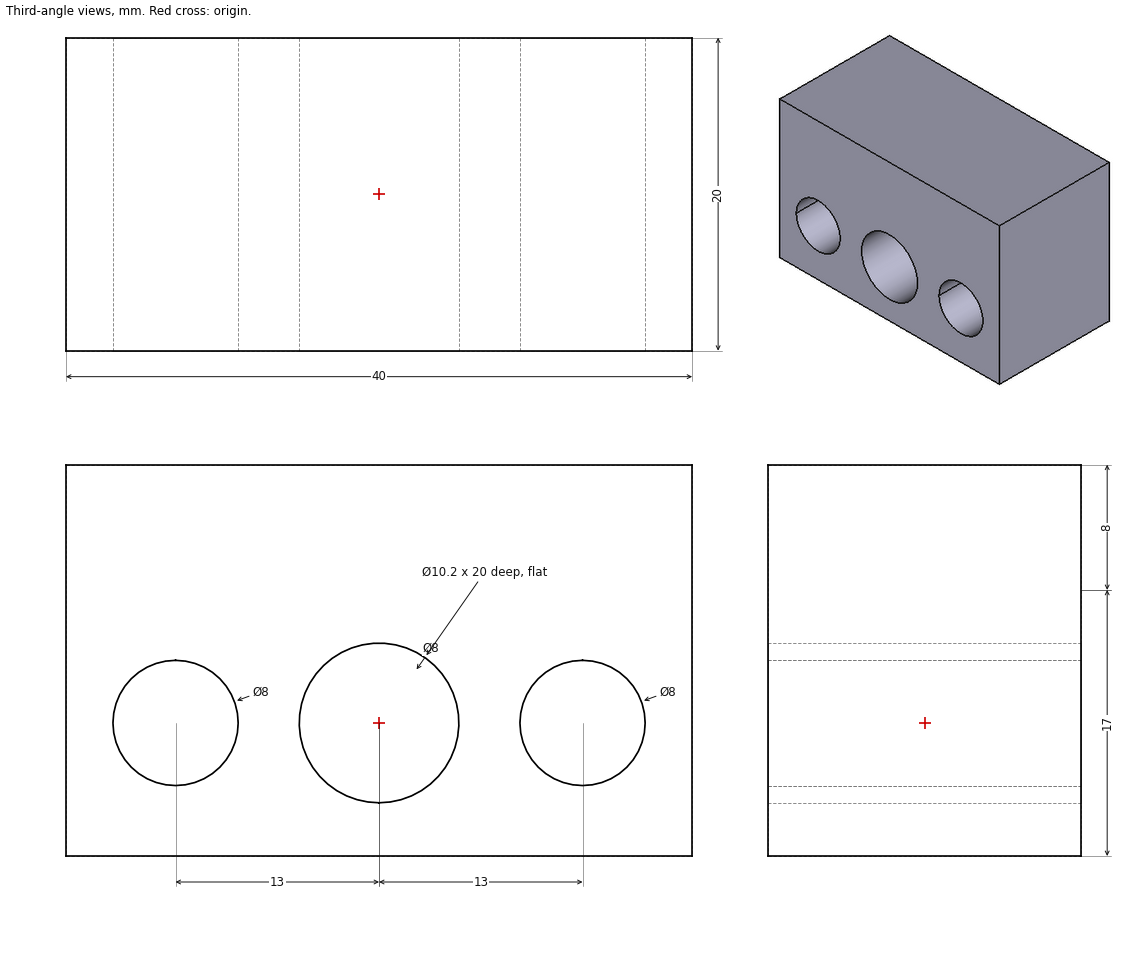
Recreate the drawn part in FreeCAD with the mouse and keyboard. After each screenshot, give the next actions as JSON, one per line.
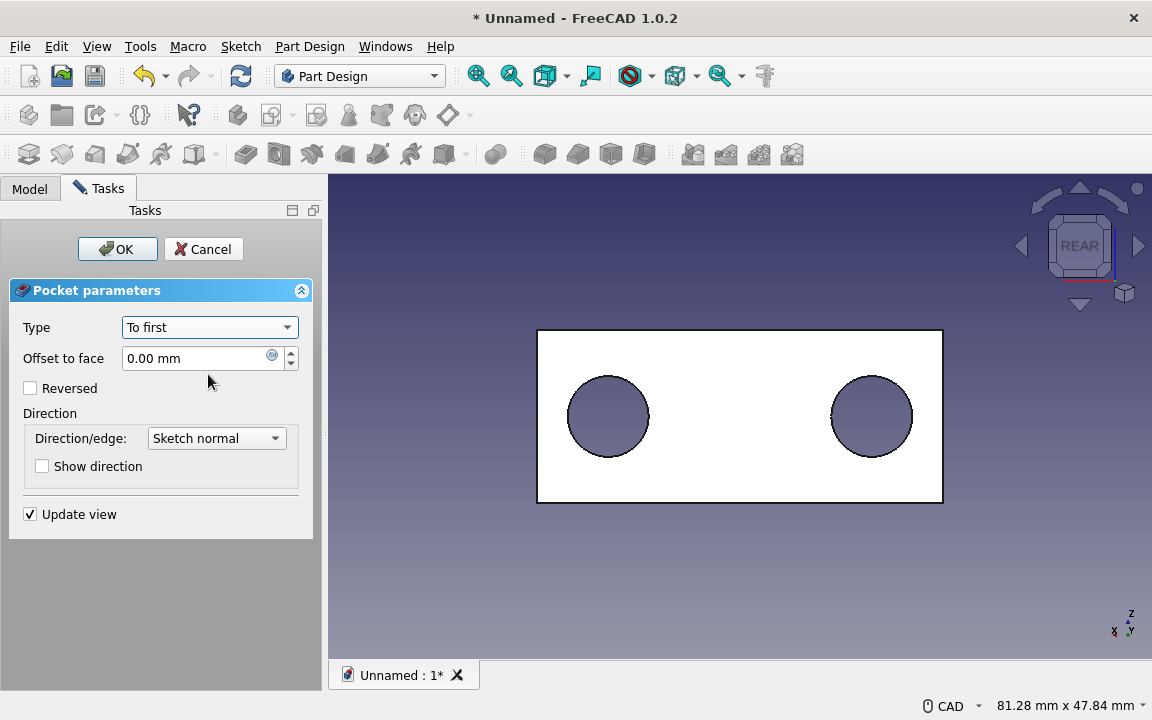
{"action": "left_click", "coordinate": [118, 249]}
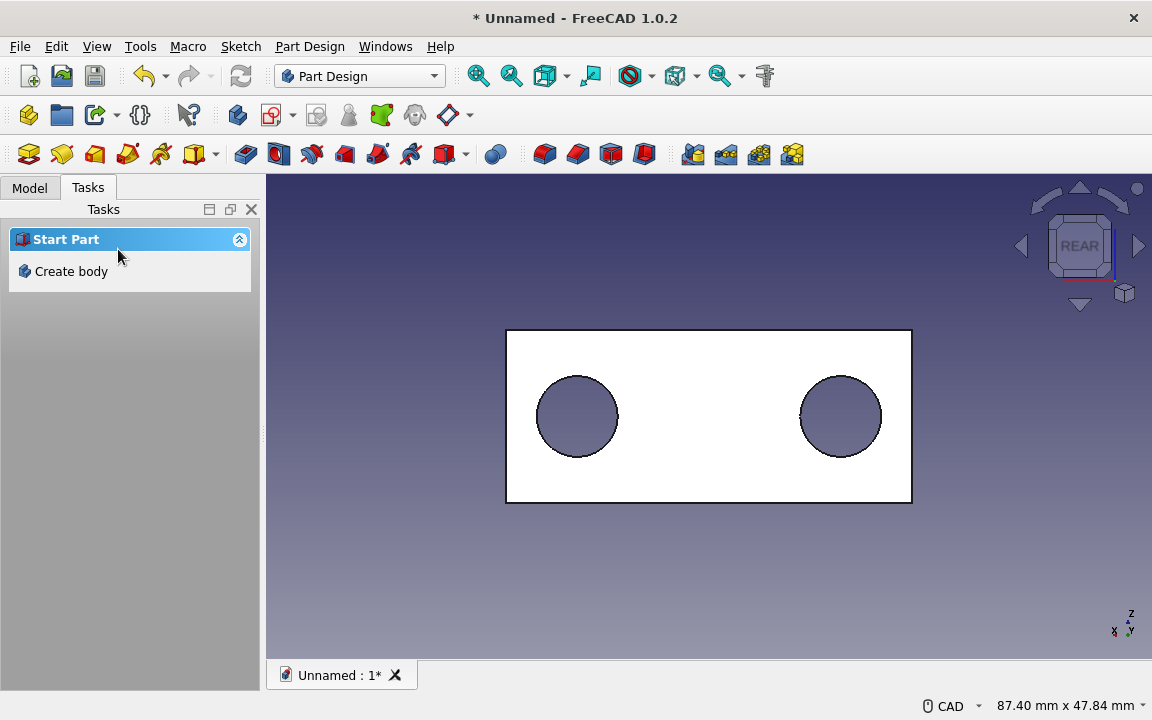
{"action": "key", "text": "0"}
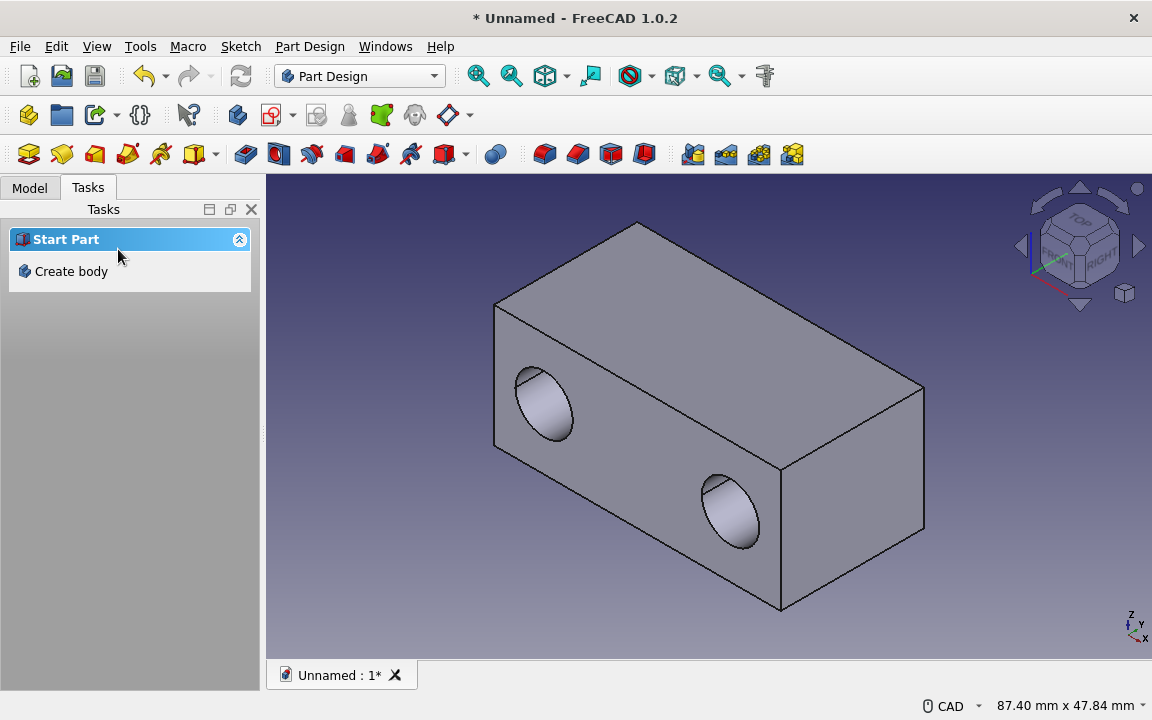
{"action": "left_click", "coordinate": [637, 457]}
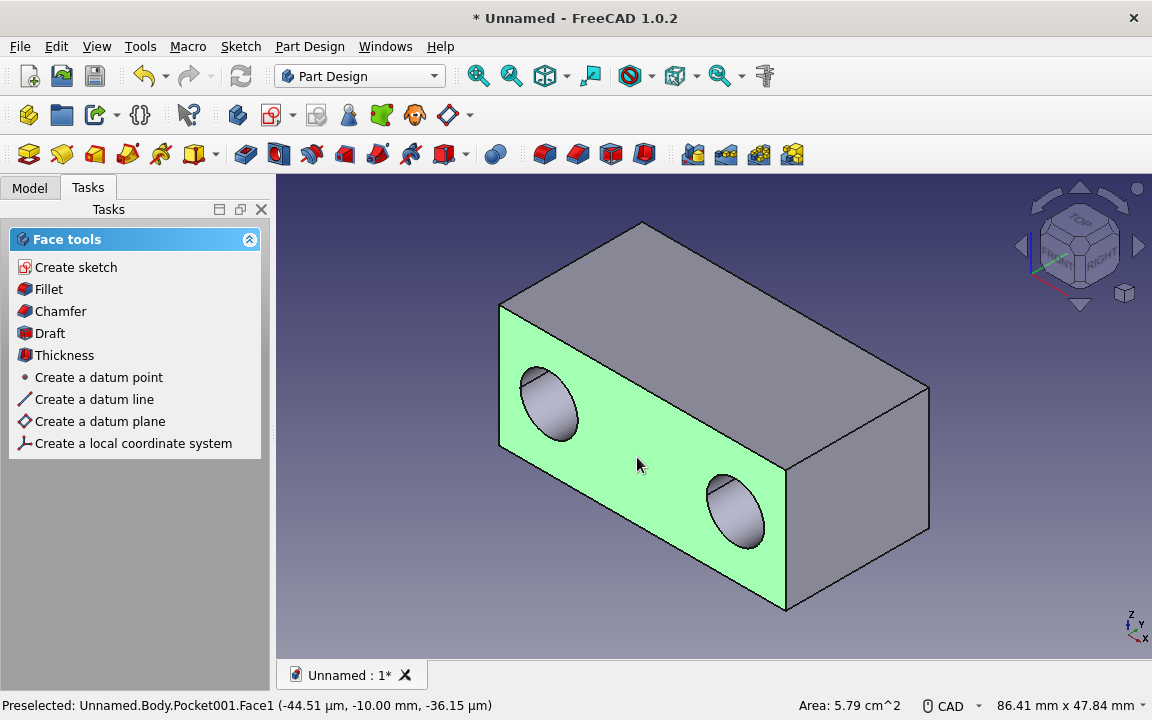
{"action": "left_click", "coordinate": [270, 116]}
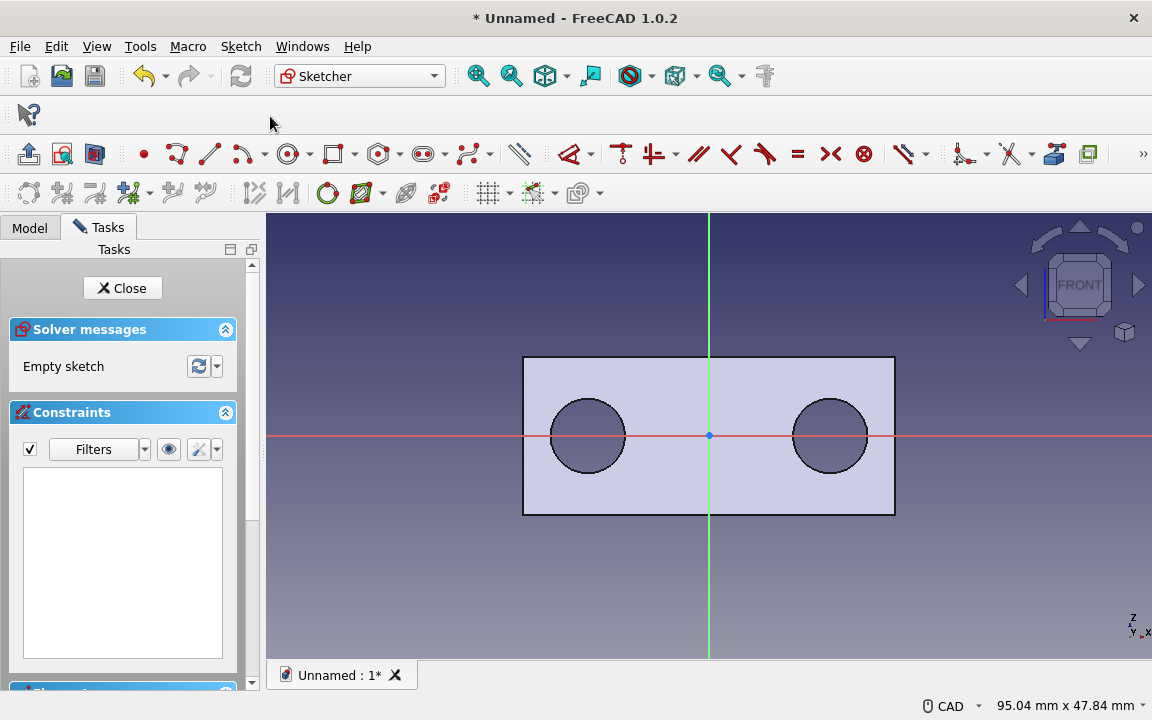
{"action": "scroll", "coordinate": [731, 436], "scroll_direction": "up", "scroll_amount": 7}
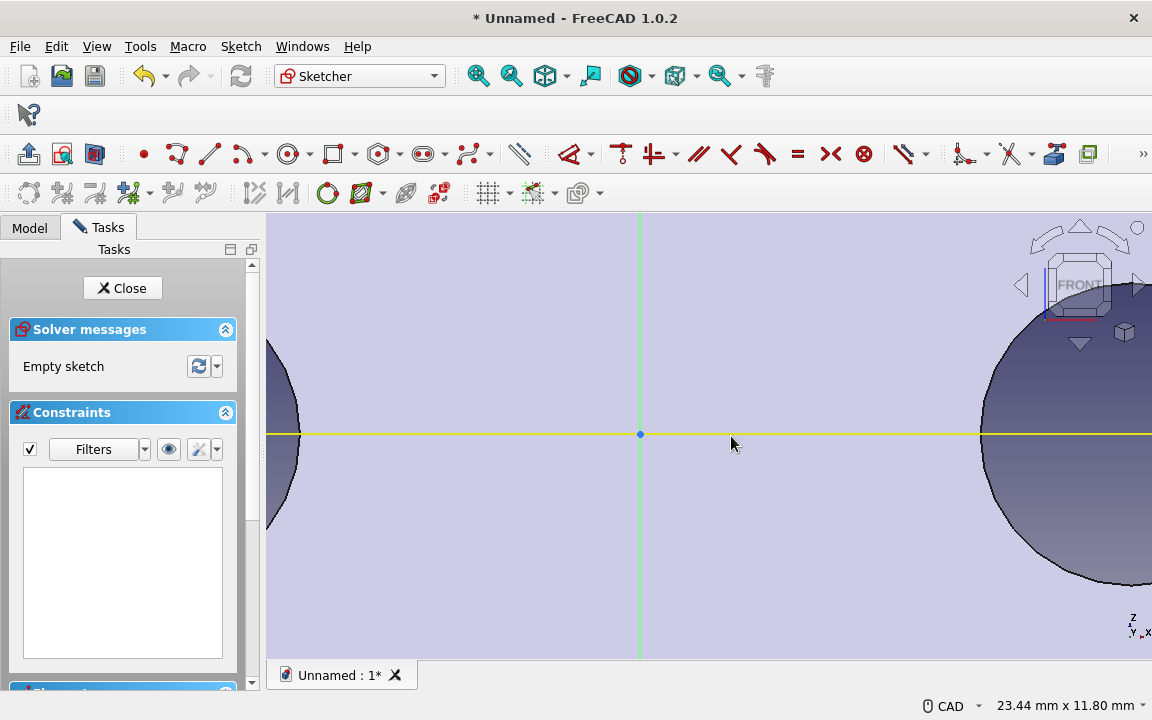
{"action": "left_click", "coordinate": [288, 154]}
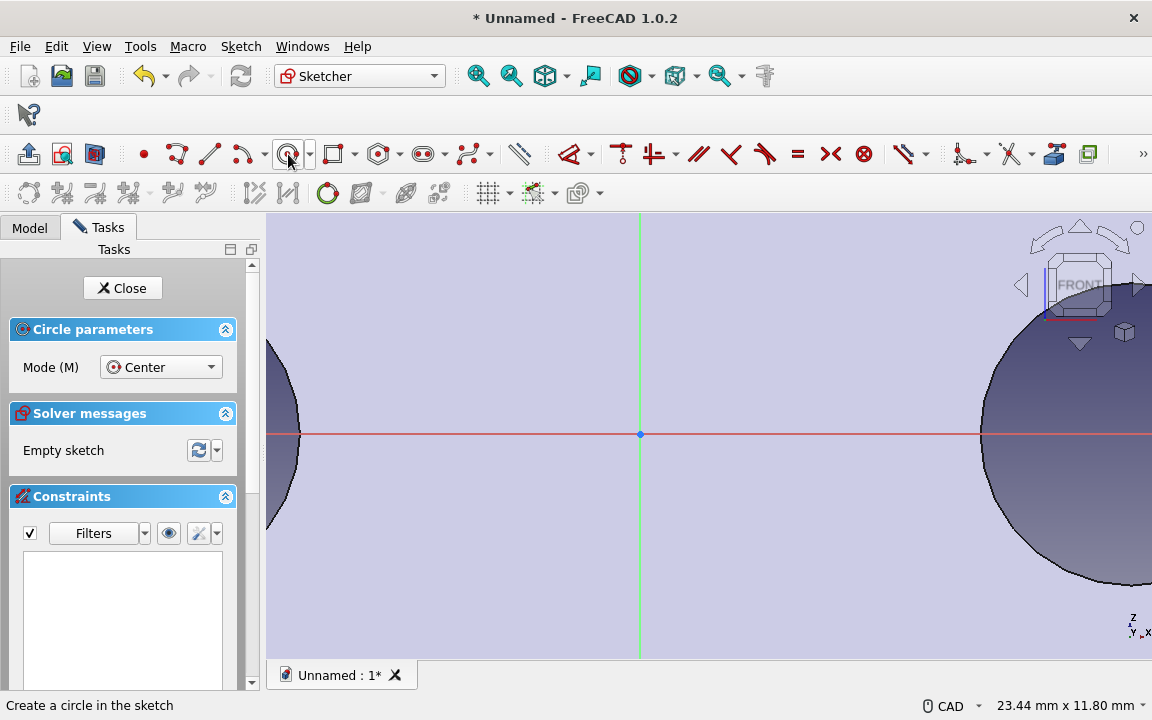
{"action": "left_click", "coordinate": [640, 434]}
{"action": "left_click", "coordinate": [747, 328]}
{"action": "key", "text": "Escape"}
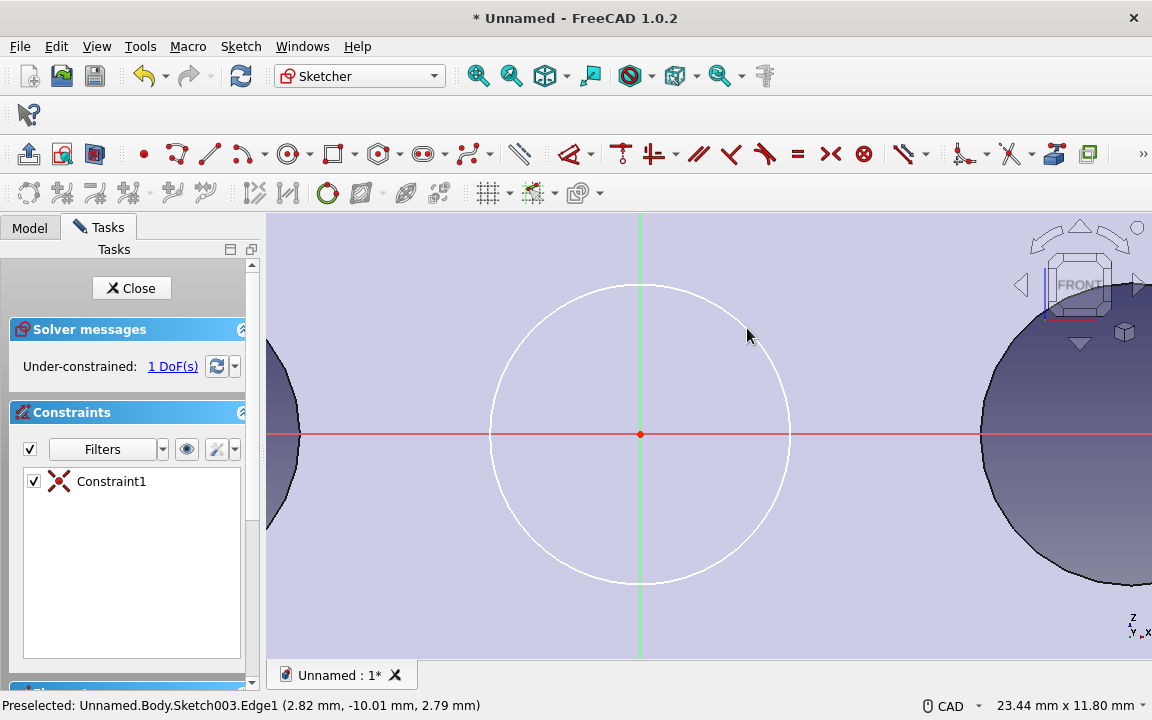
{"action": "left_click", "coordinate": [568, 154]}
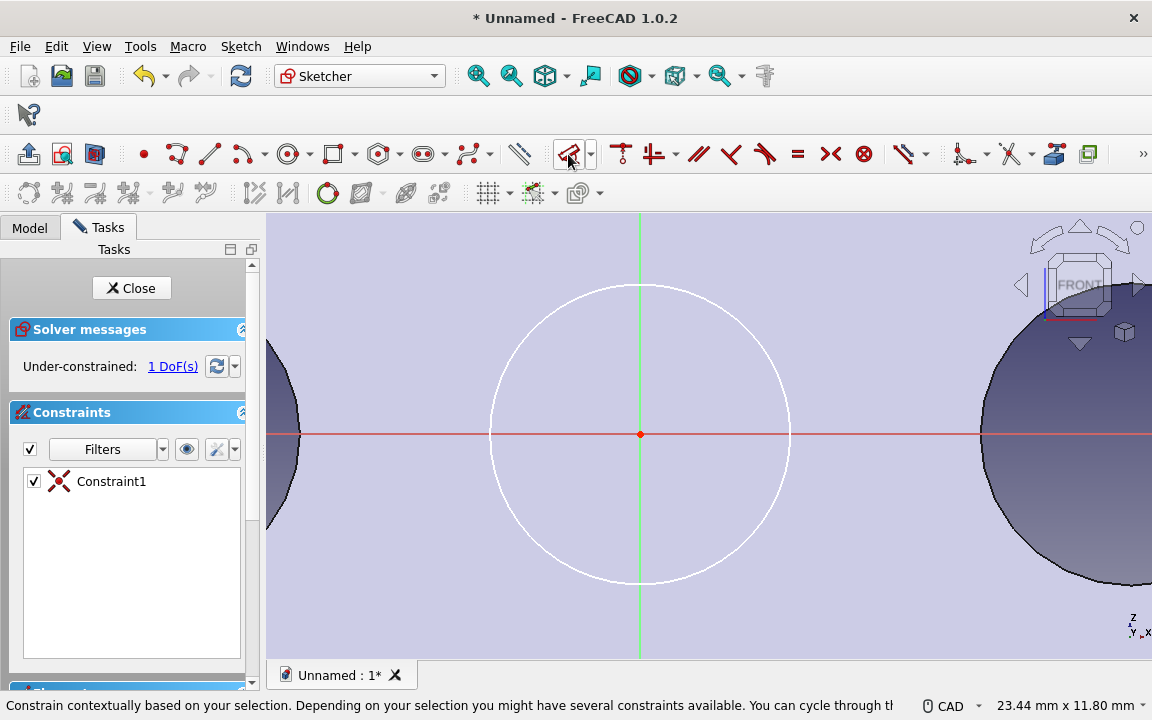
{"action": "left_click", "coordinate": [746, 328]}
{"action": "left_click", "coordinate": [769, 305]}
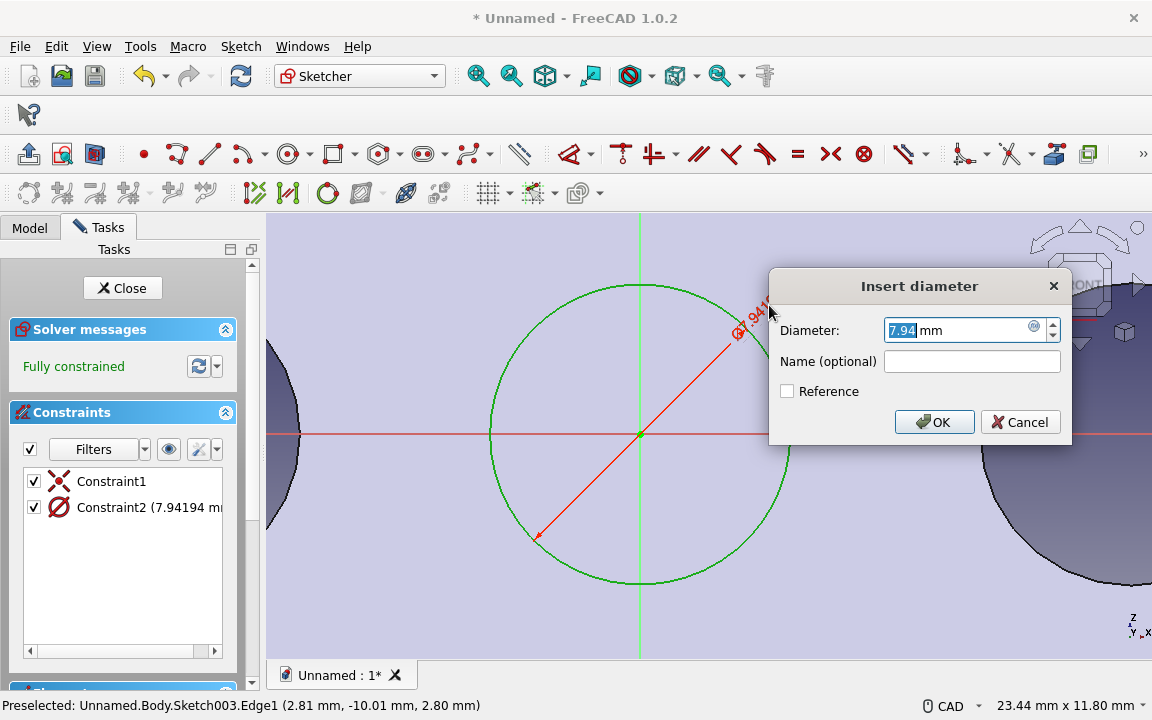
{"action": "type", "text": "8"}
{"action": "key", "text": "Return"}
{"action": "key", "text": "Escape"}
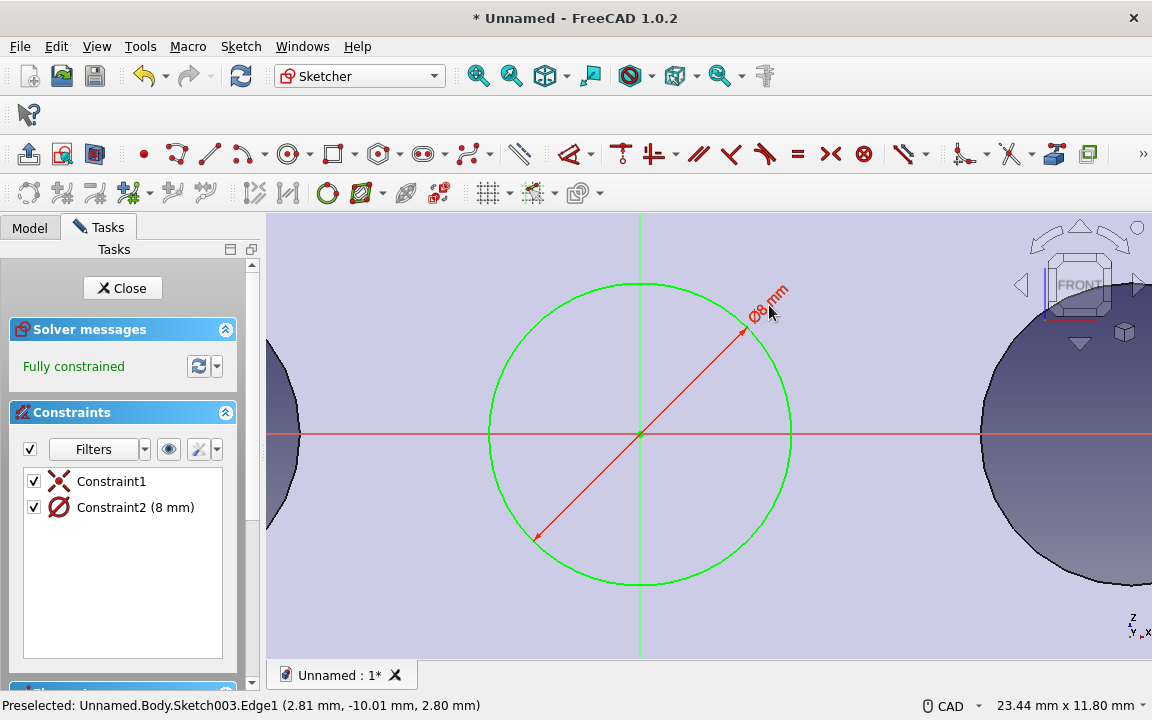
{"action": "left_click", "coordinate": [123, 288]}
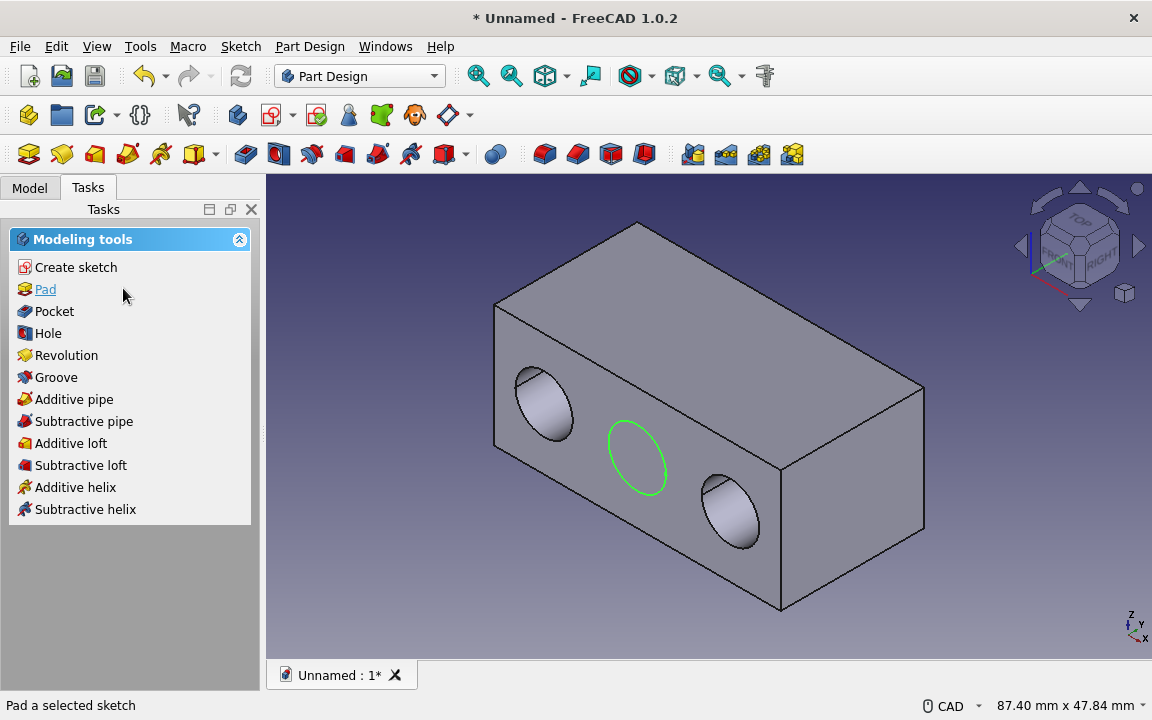
{"action": "left_click", "coordinate": [246, 154]}